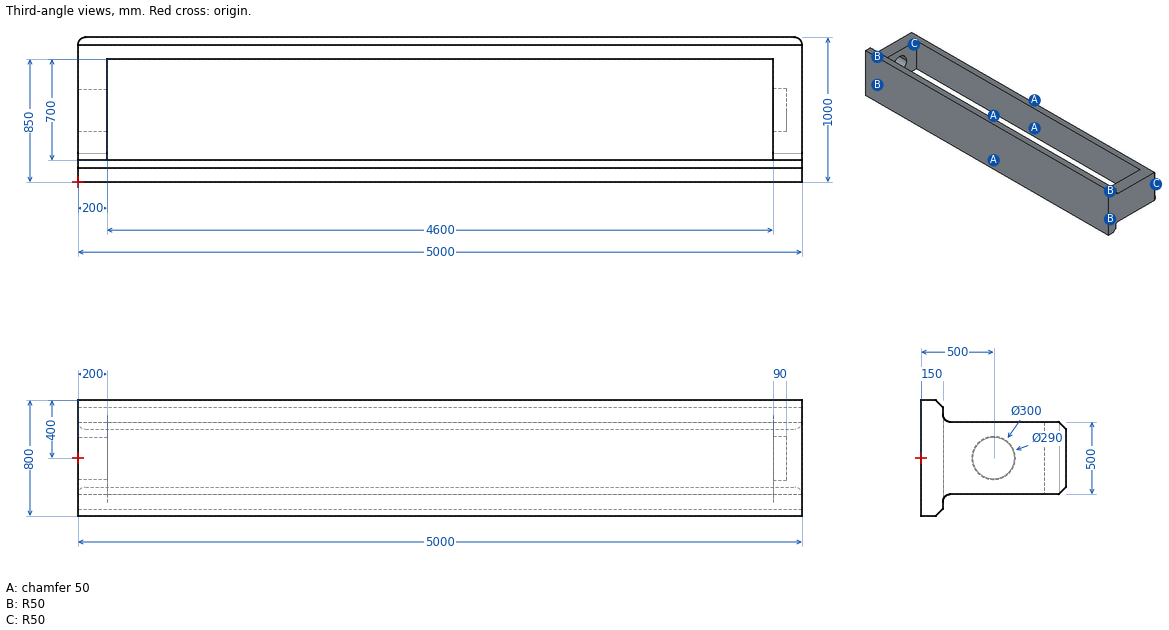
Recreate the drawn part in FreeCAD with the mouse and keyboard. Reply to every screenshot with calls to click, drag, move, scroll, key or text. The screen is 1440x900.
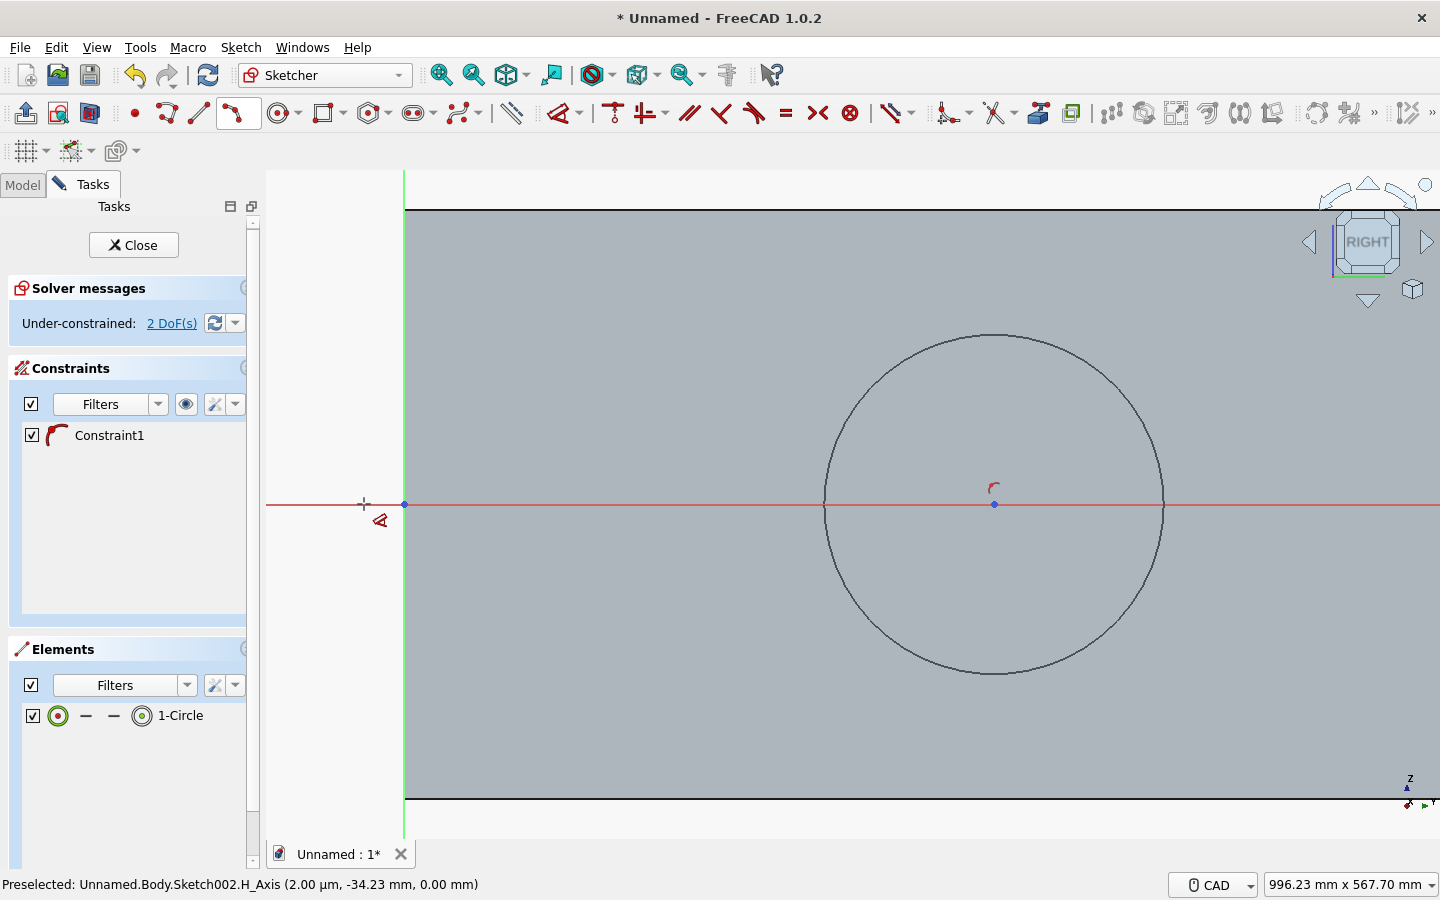
click(1114, 384)
click(1137, 361)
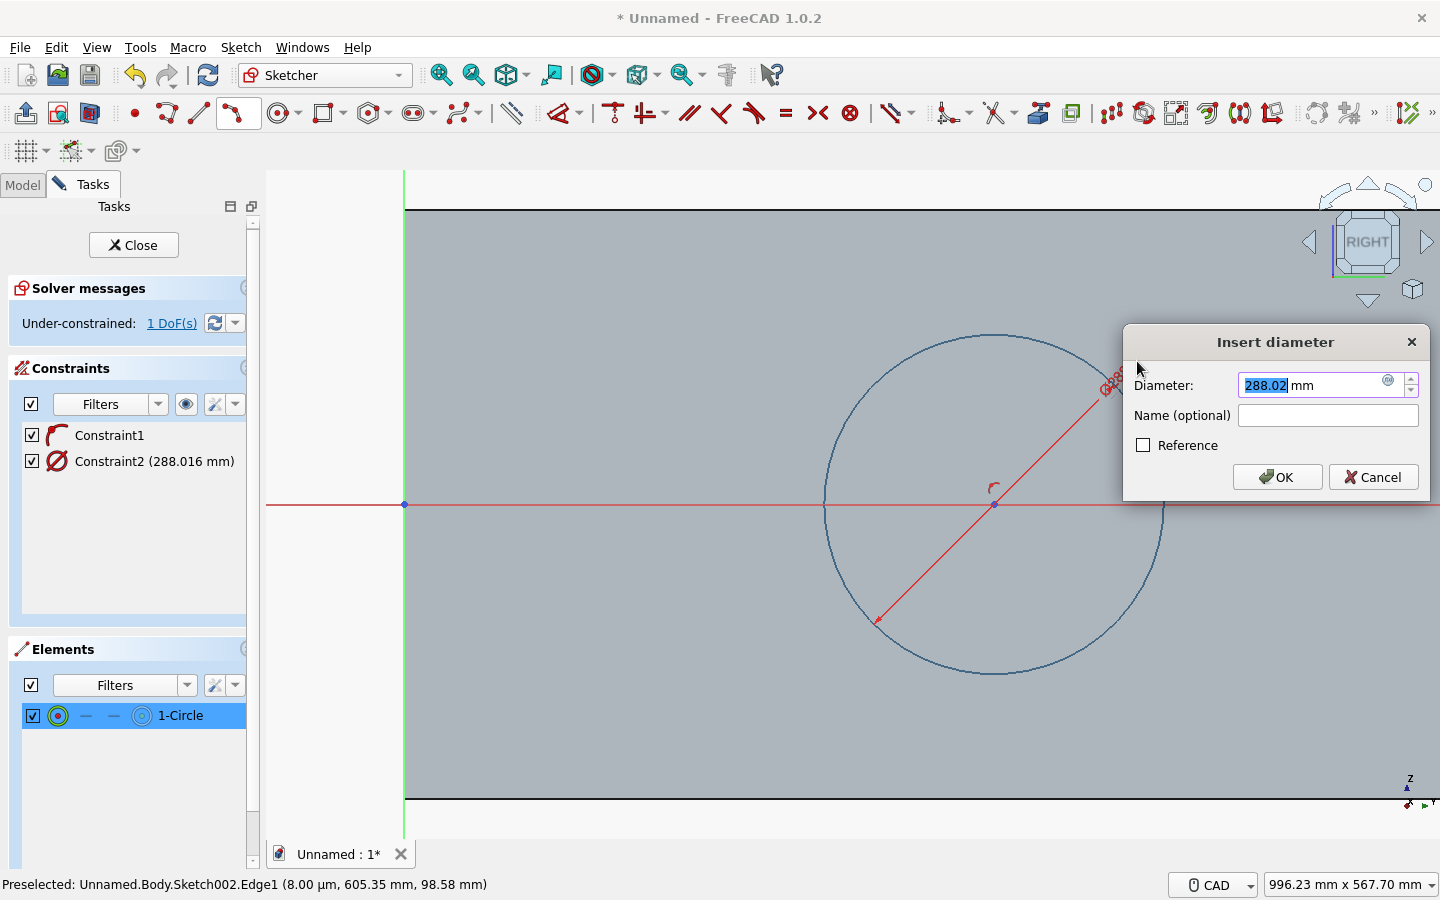
text(290)
key(Return)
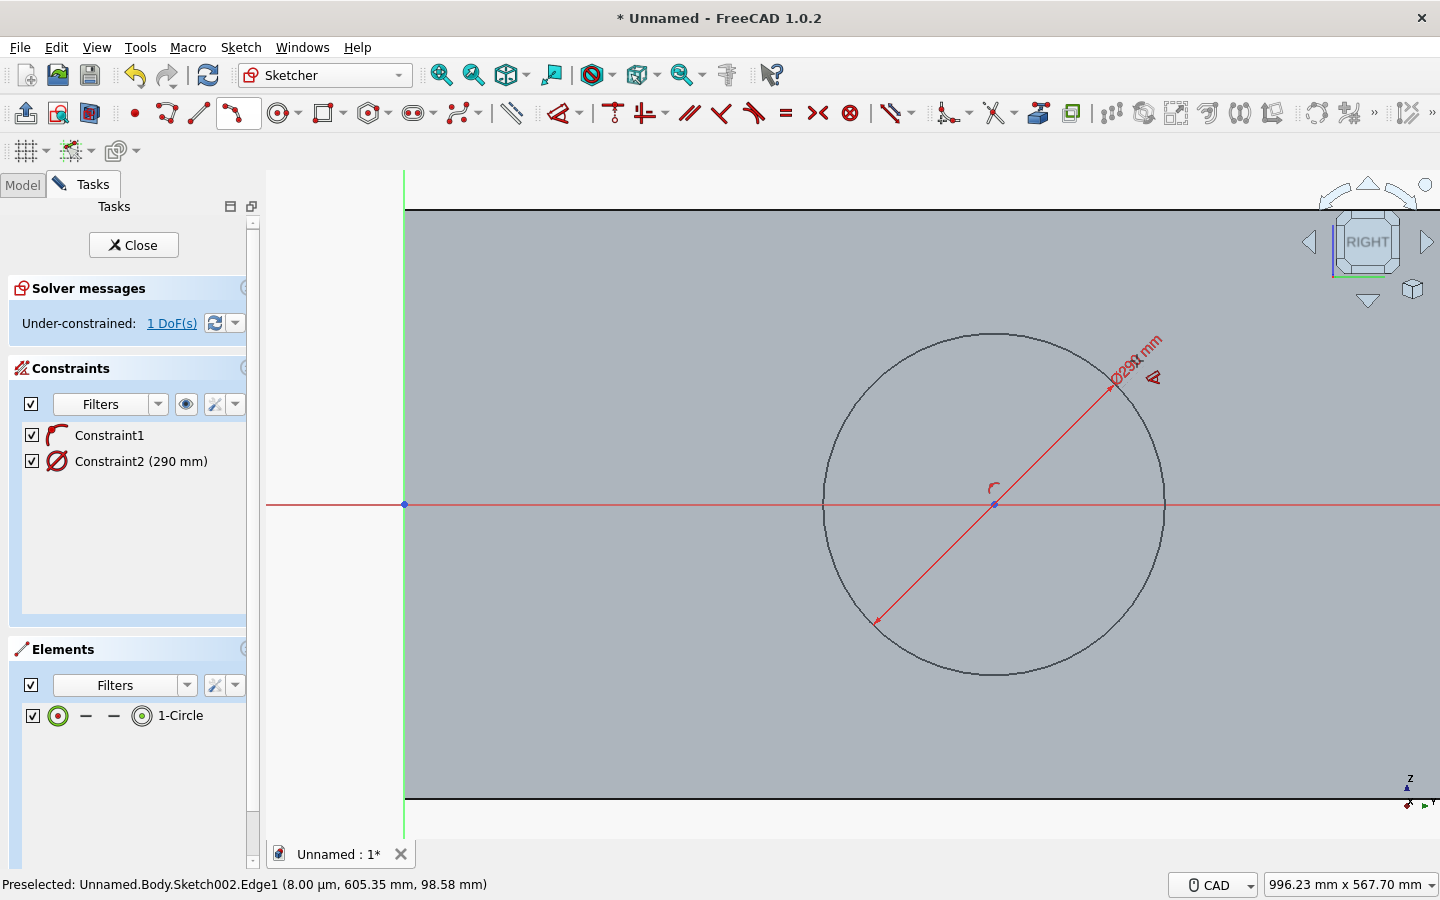
click(994, 504)
click(699, 538)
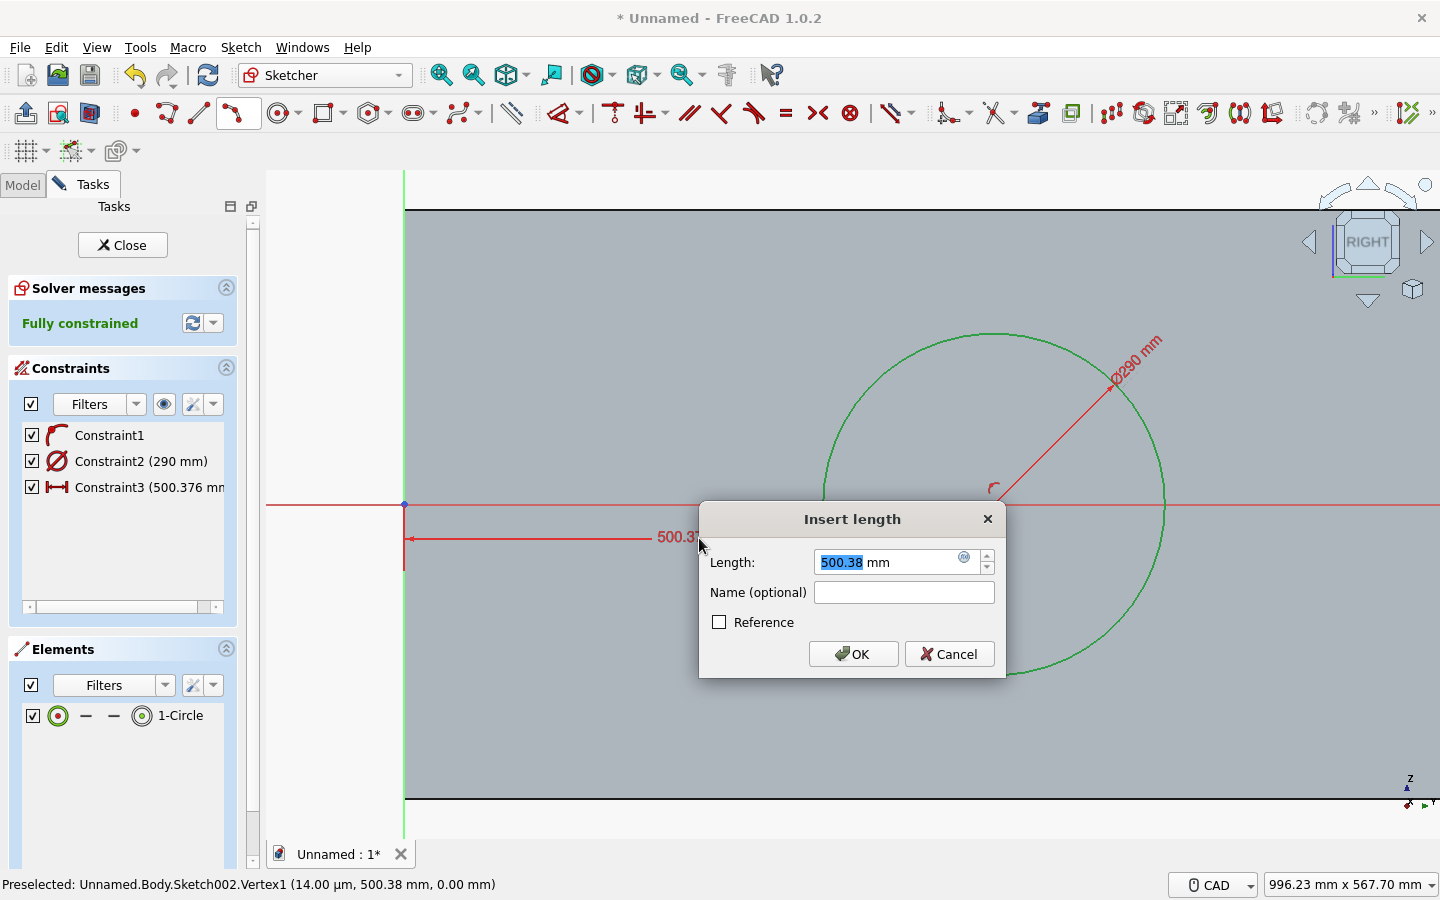
text(500)
key(Return)
key(Escape)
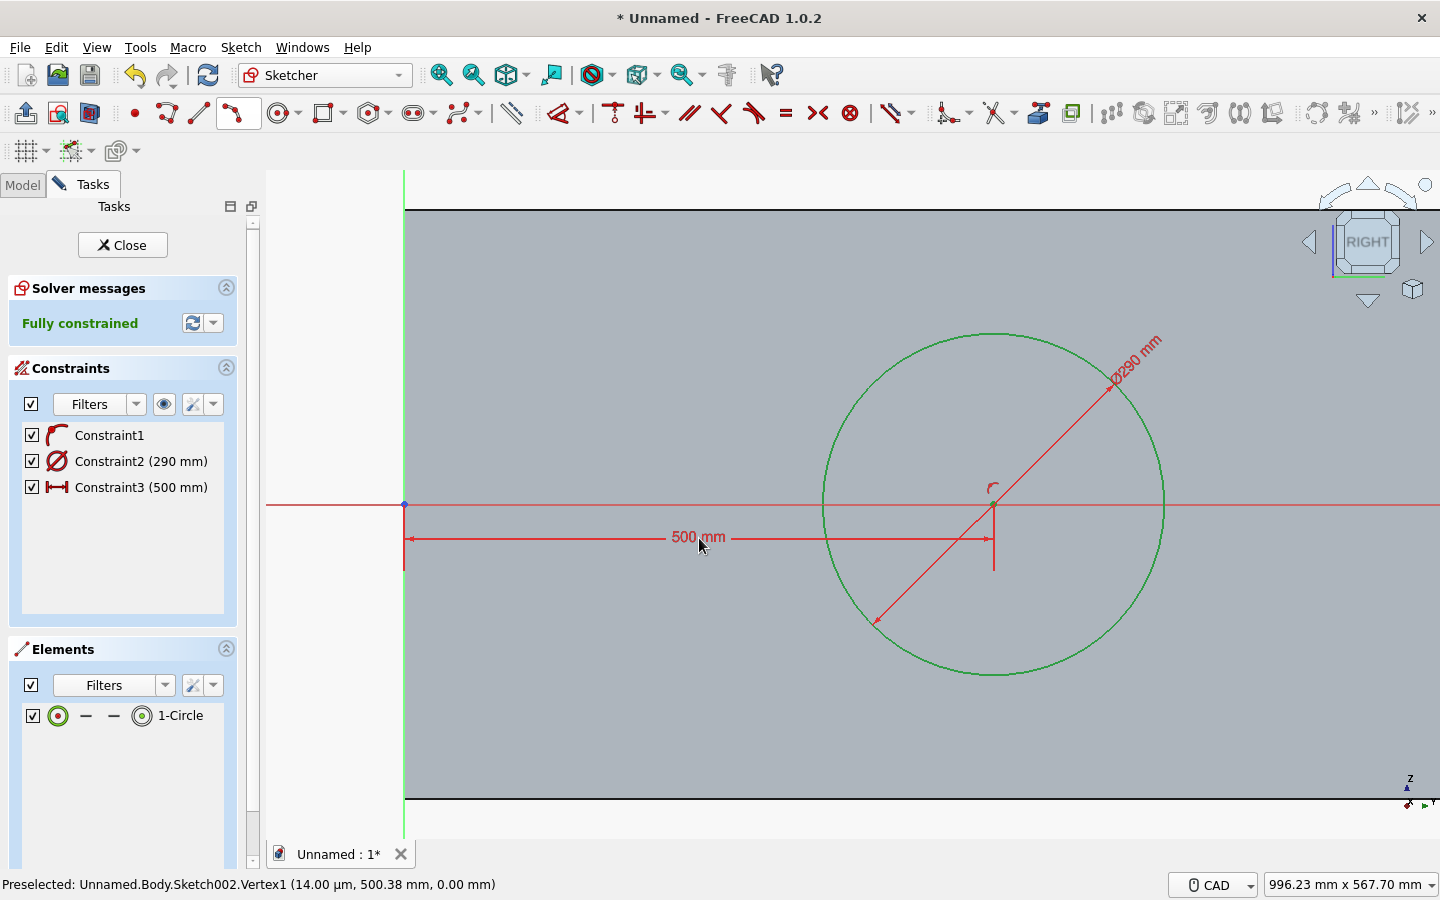
click(123, 245)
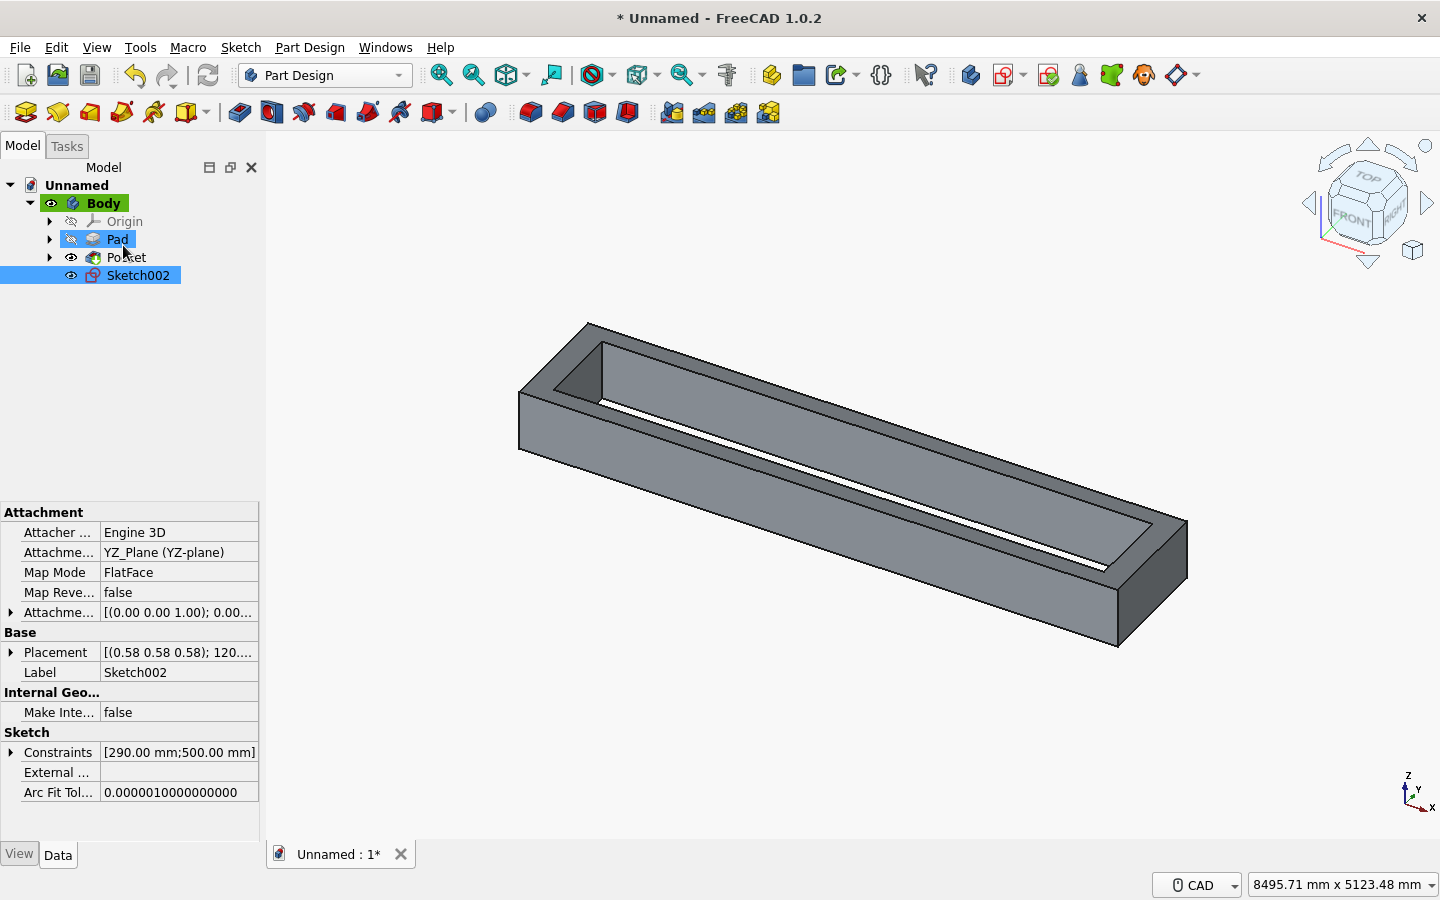
click(240, 112)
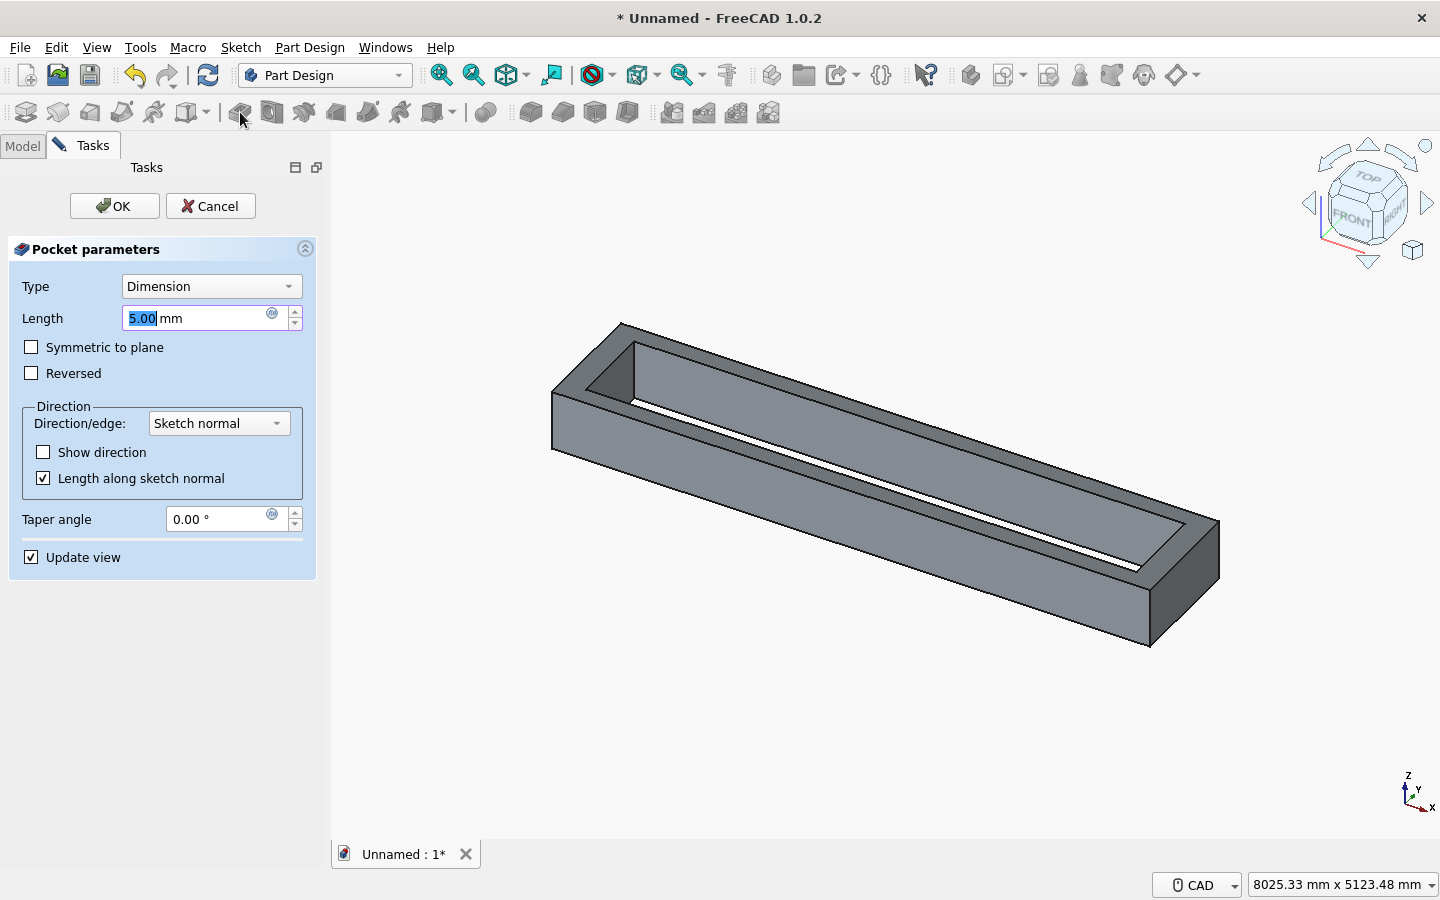
click(212, 286)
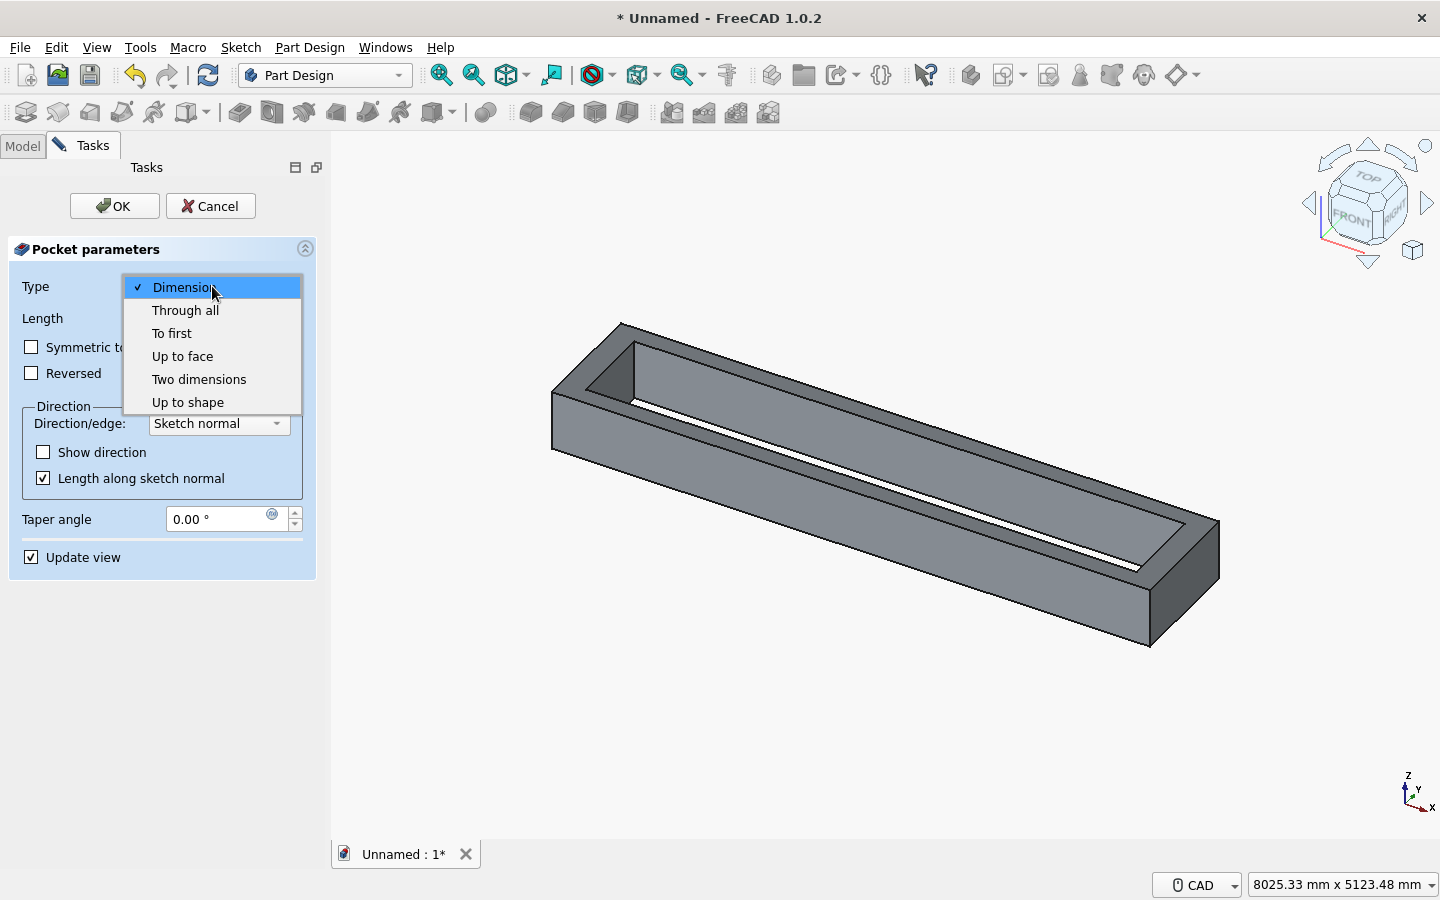
click(212, 380)